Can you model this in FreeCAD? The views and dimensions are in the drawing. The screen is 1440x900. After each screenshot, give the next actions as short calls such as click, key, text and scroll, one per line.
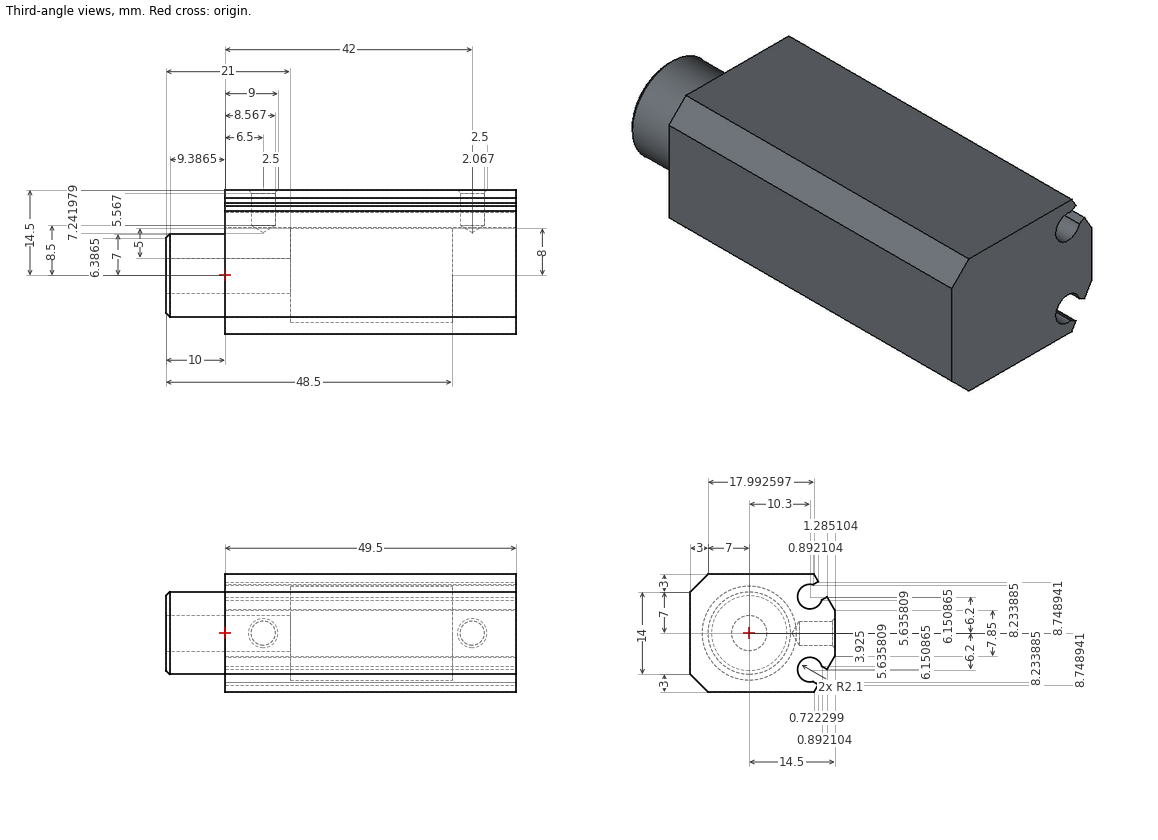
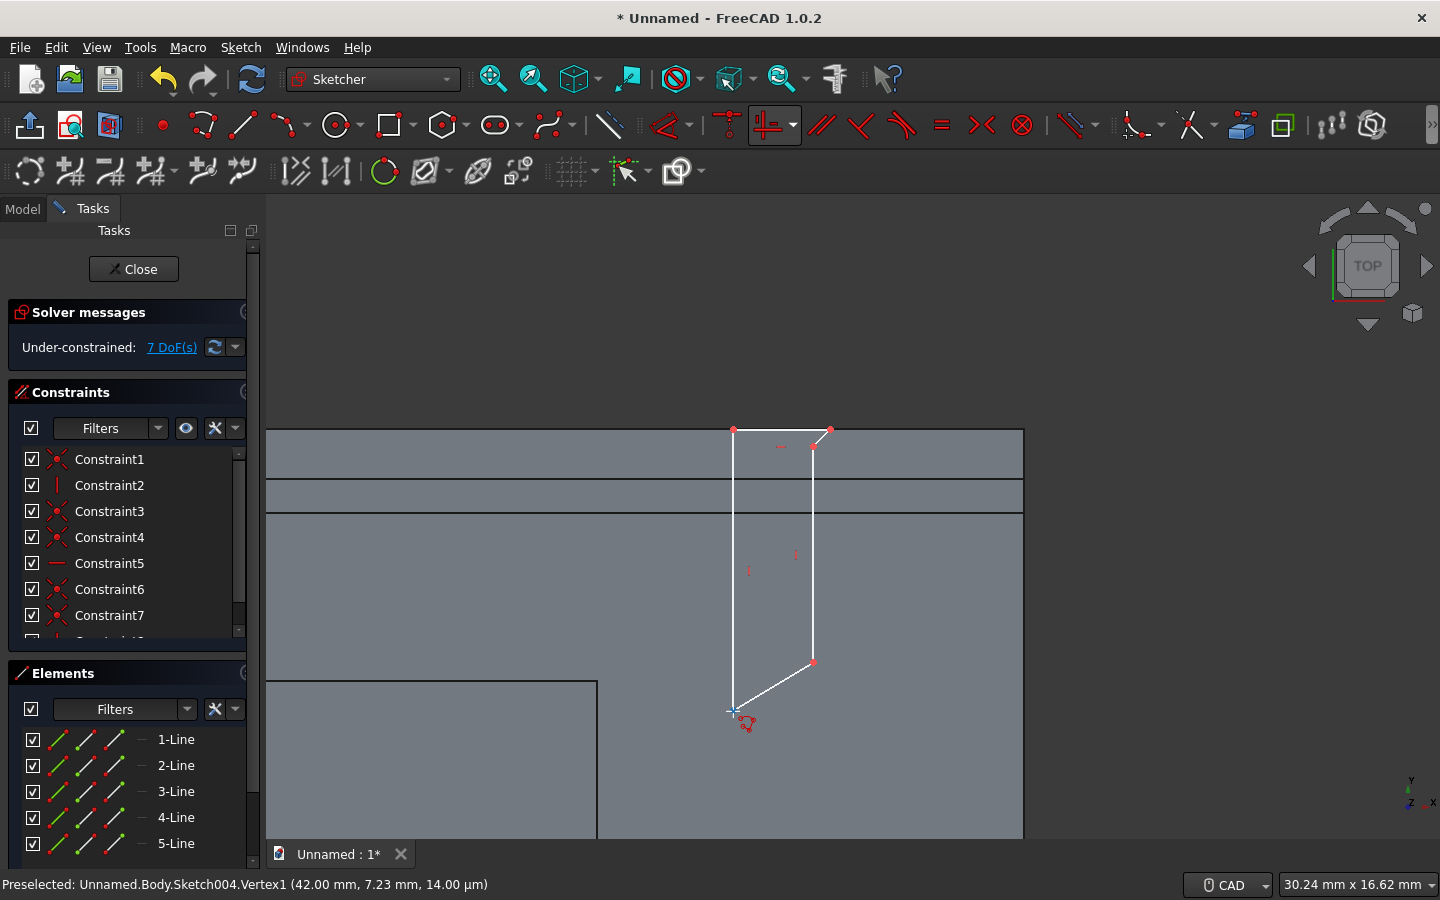
click(244, 126)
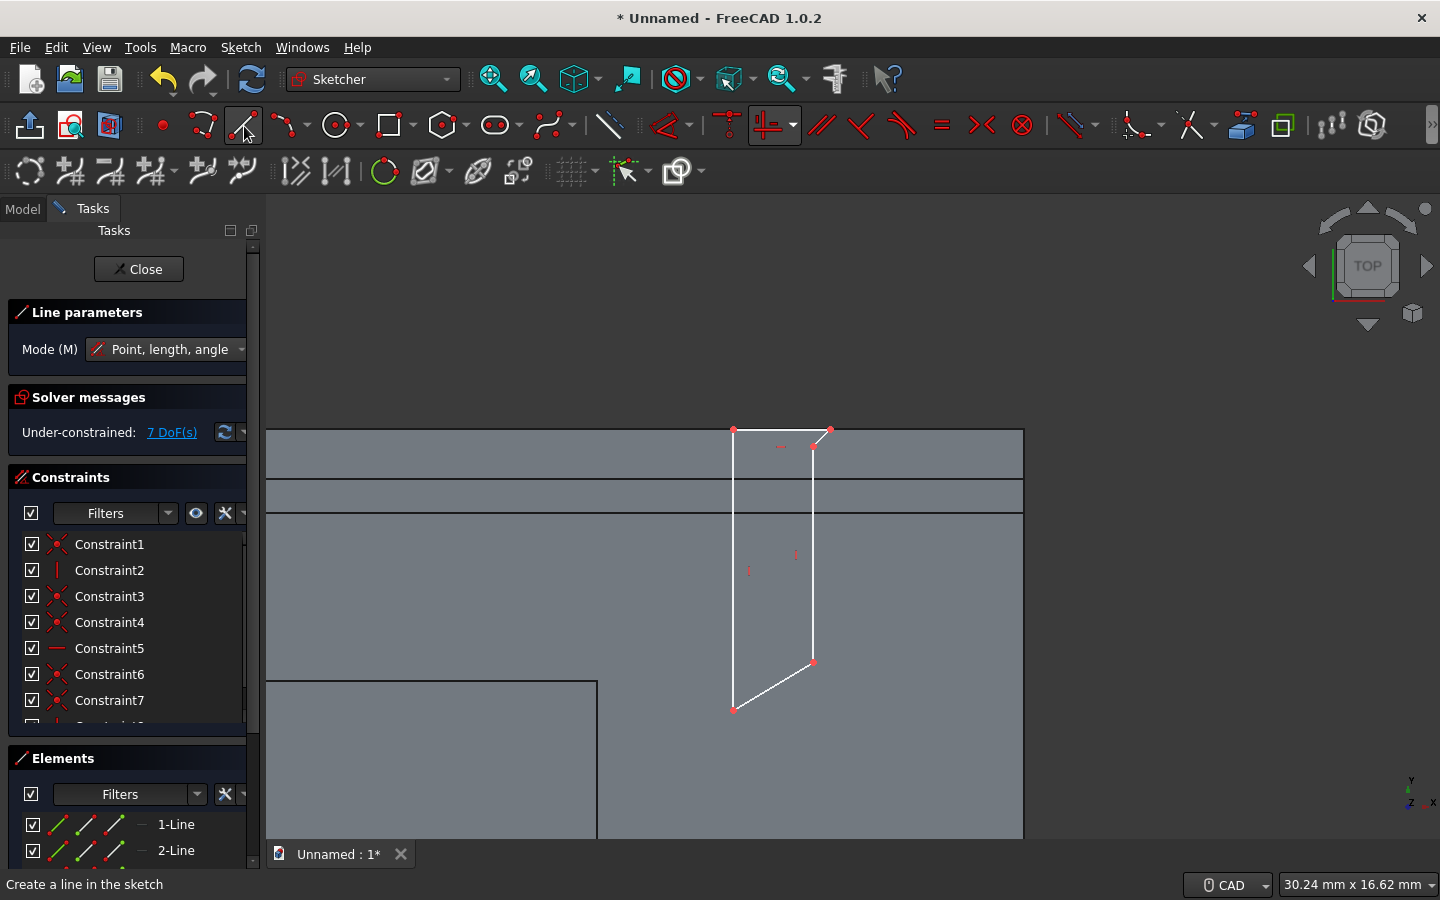
click(733, 401)
click(733, 317)
key(Escape)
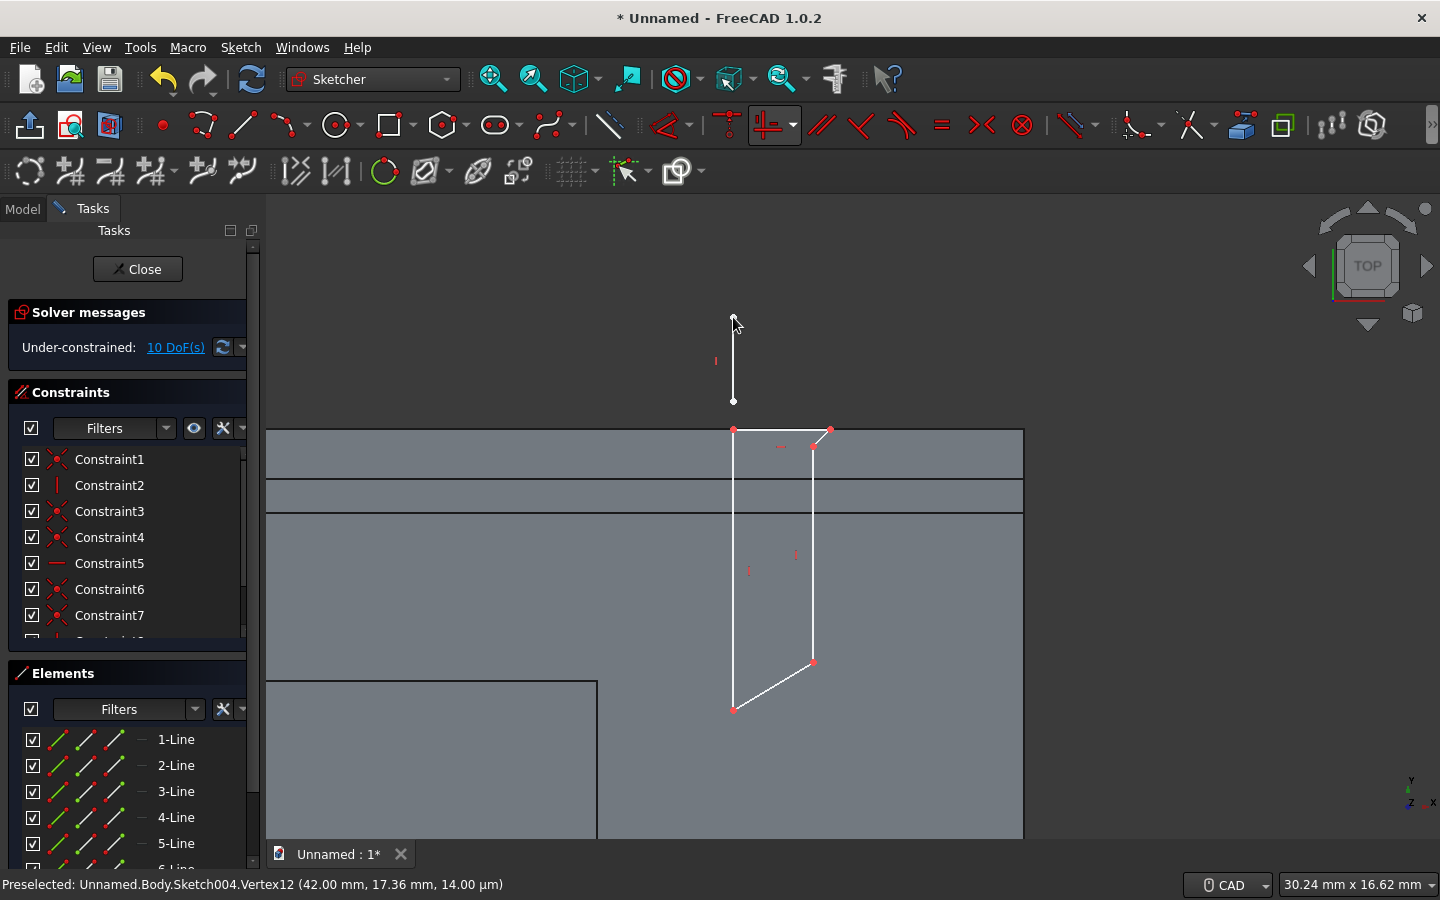
click(733, 377)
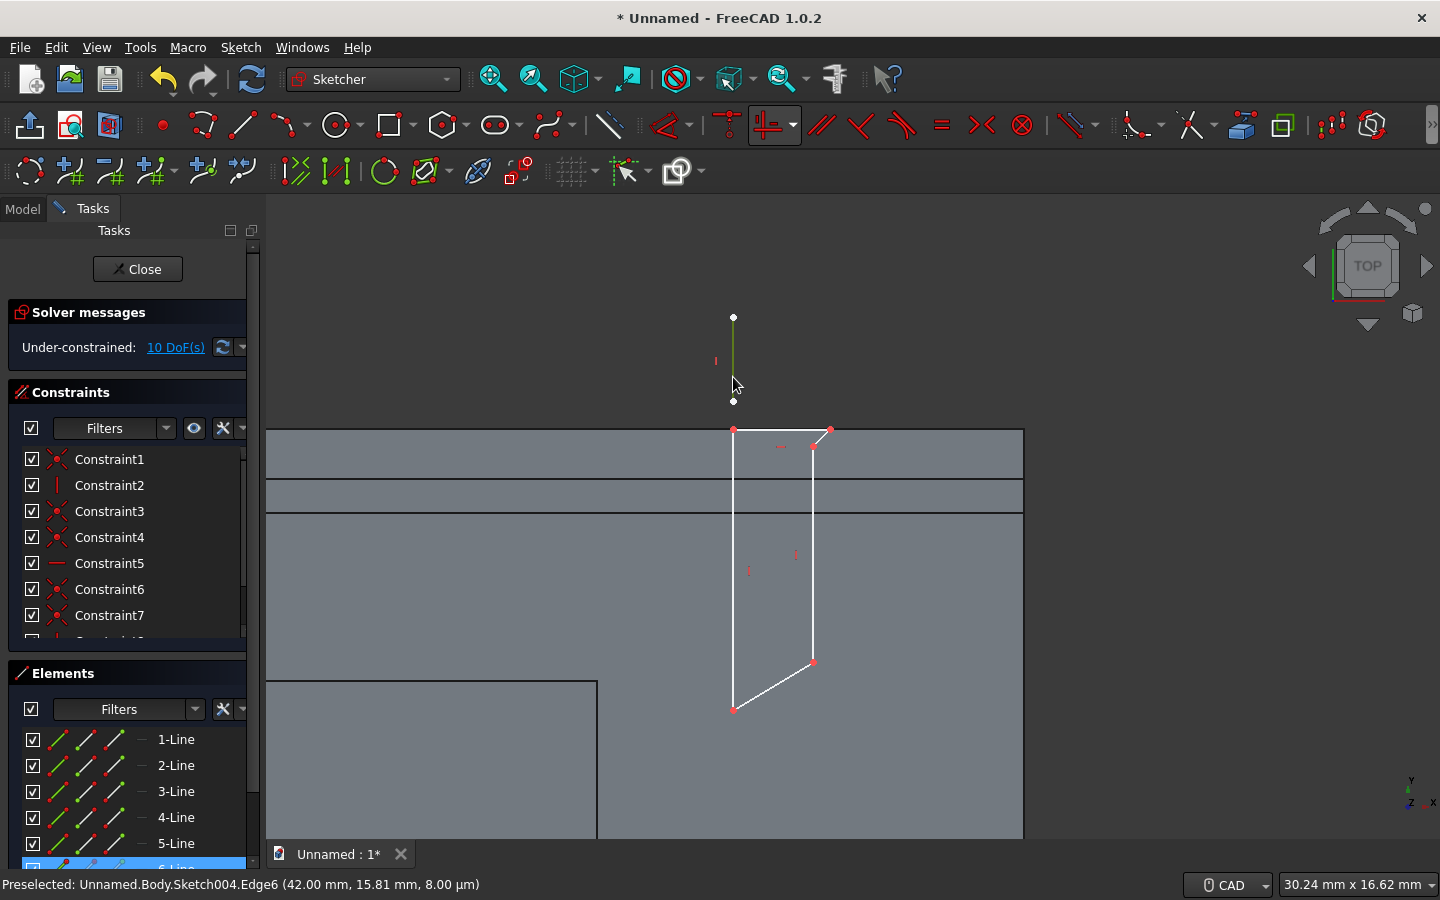
key(g)
key(n)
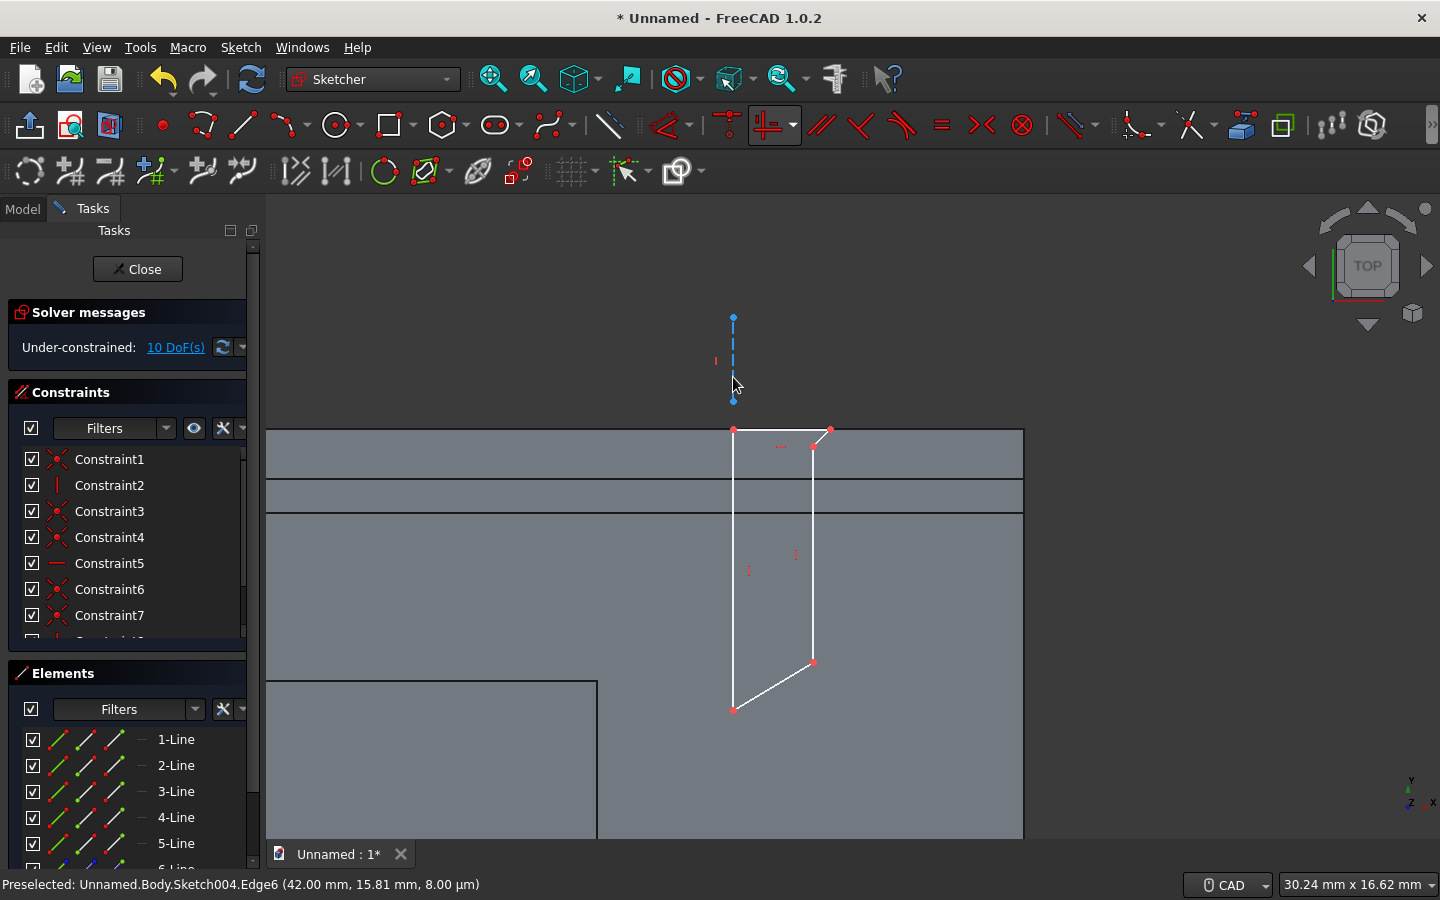
click(664, 126)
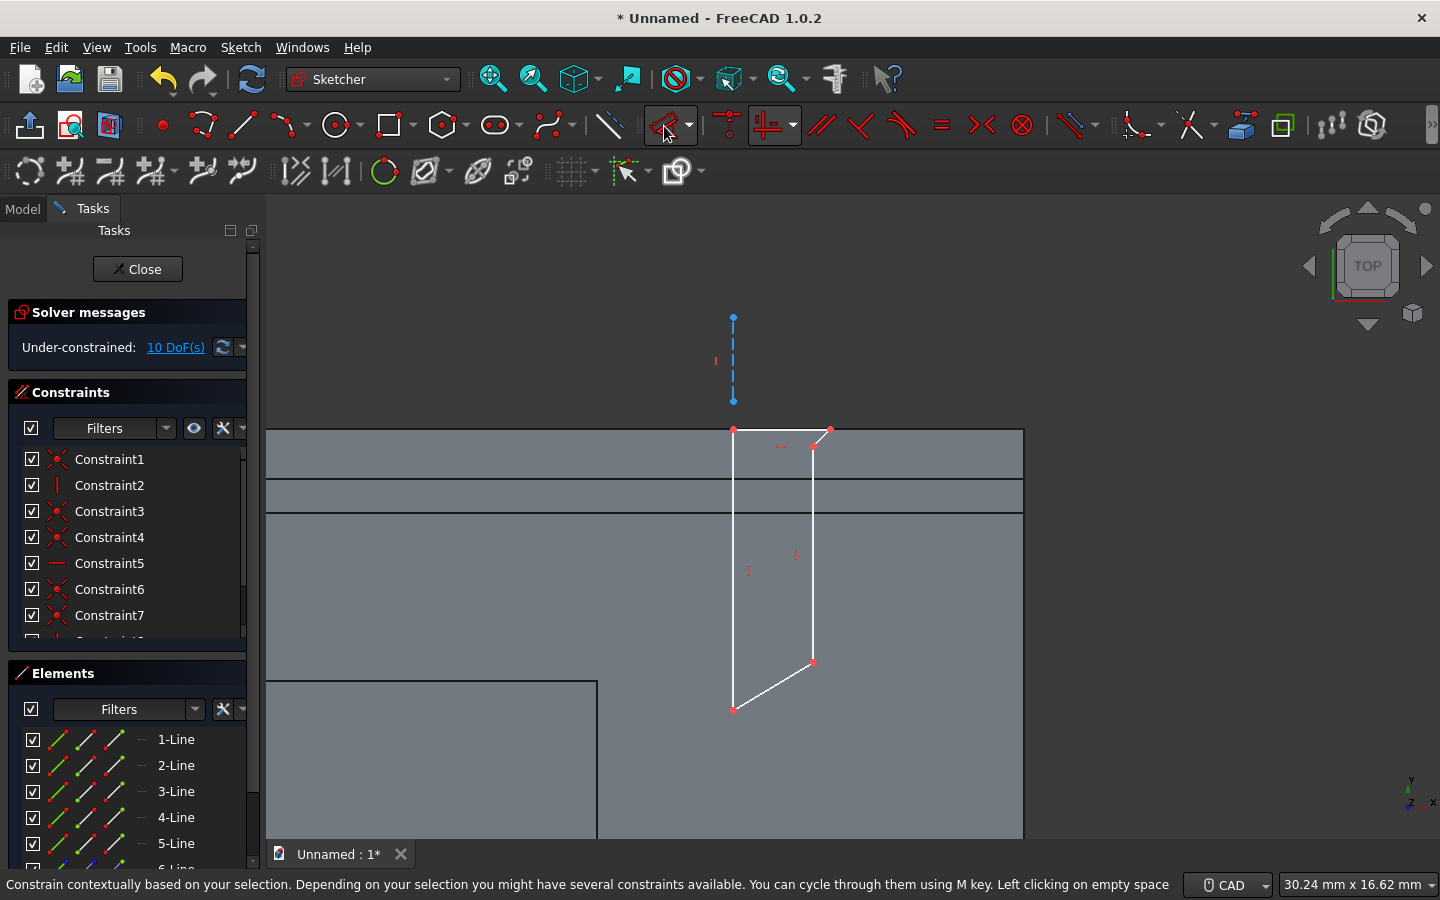
click(801, 430)
click(782, 396)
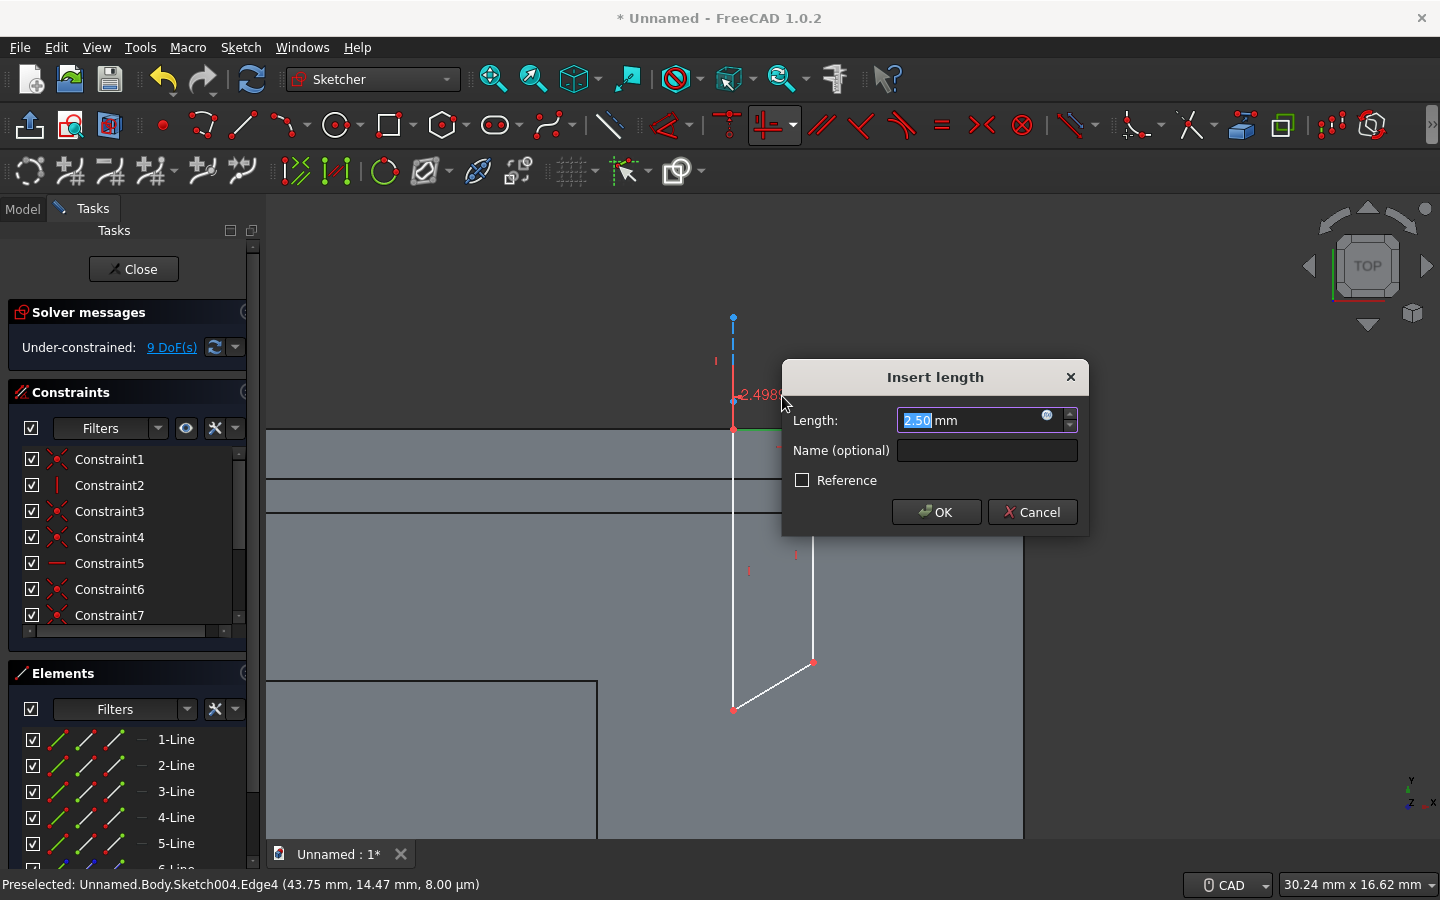
text(2.5)
key(Return)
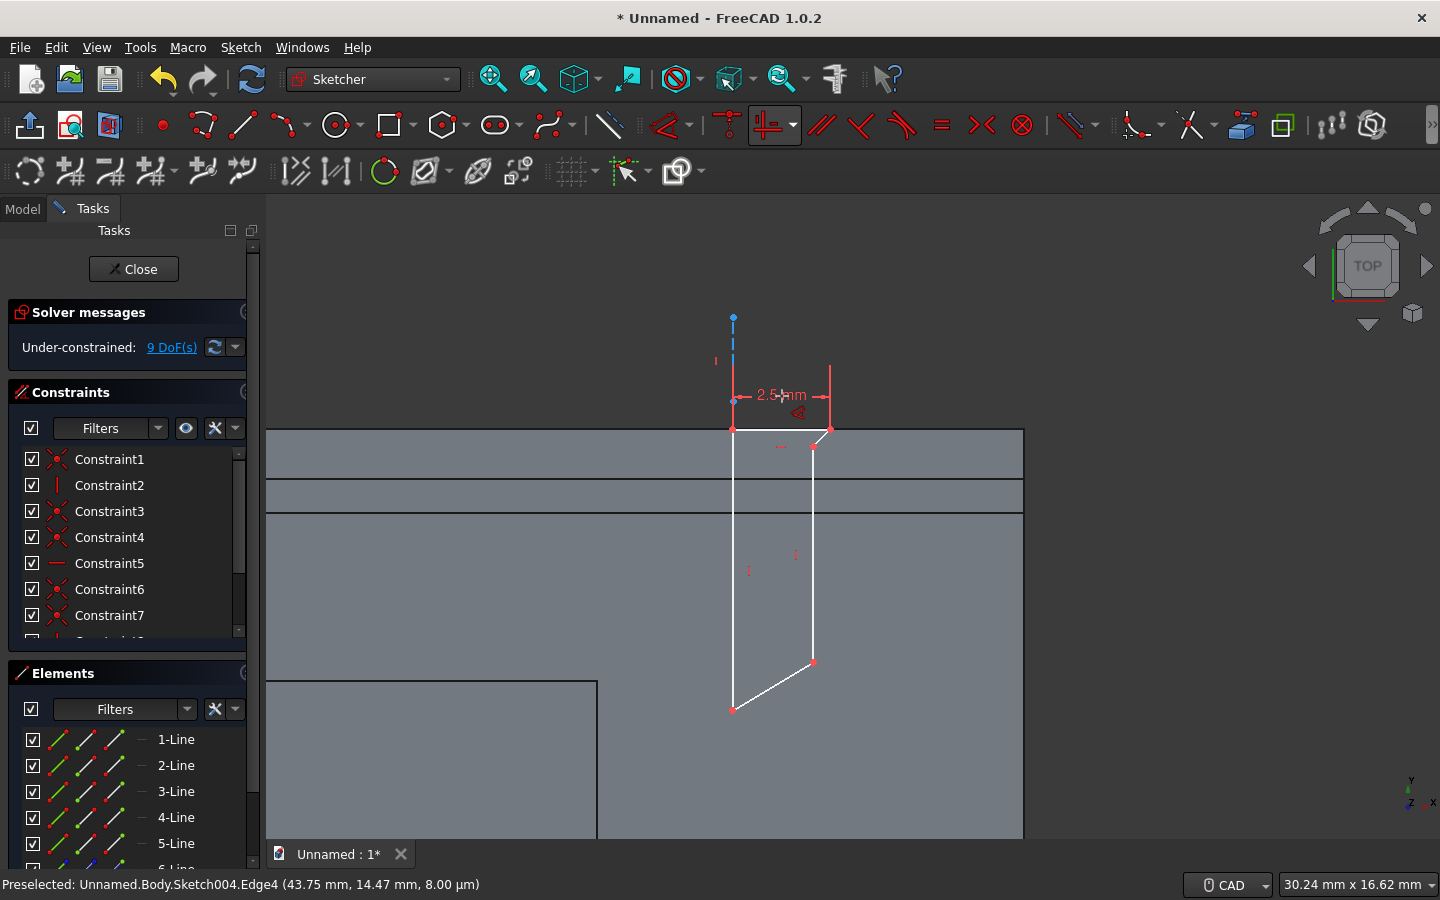
click(733, 711)
click(513, 677)